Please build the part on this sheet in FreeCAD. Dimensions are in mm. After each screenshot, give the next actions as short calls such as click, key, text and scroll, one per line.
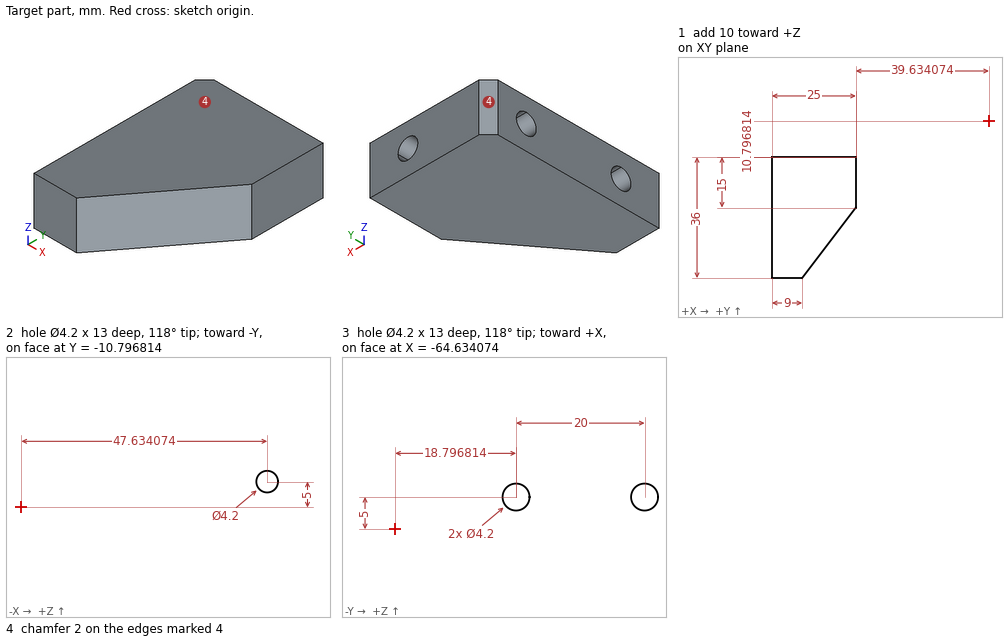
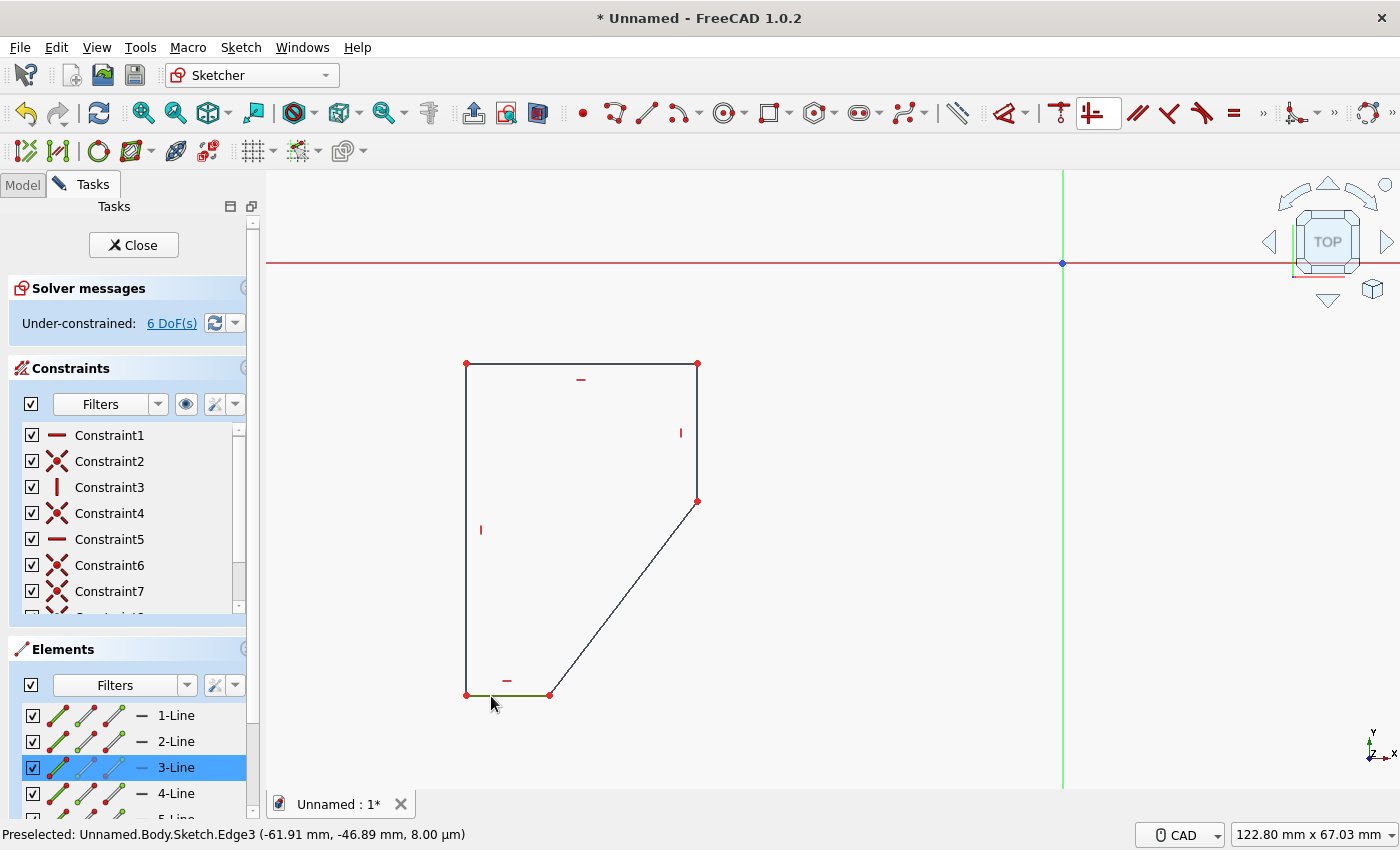
click(1028, 114)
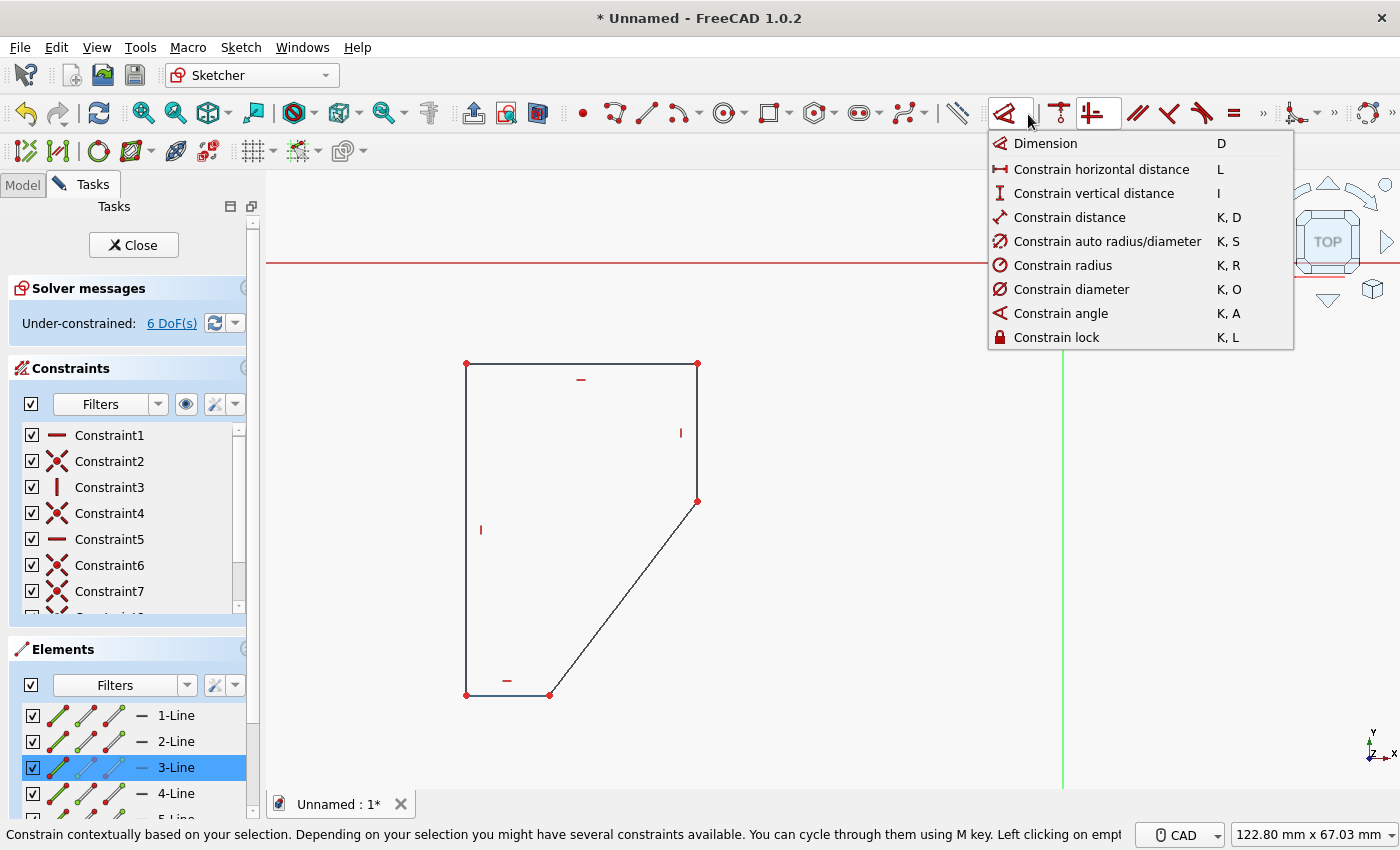
click(1141, 169)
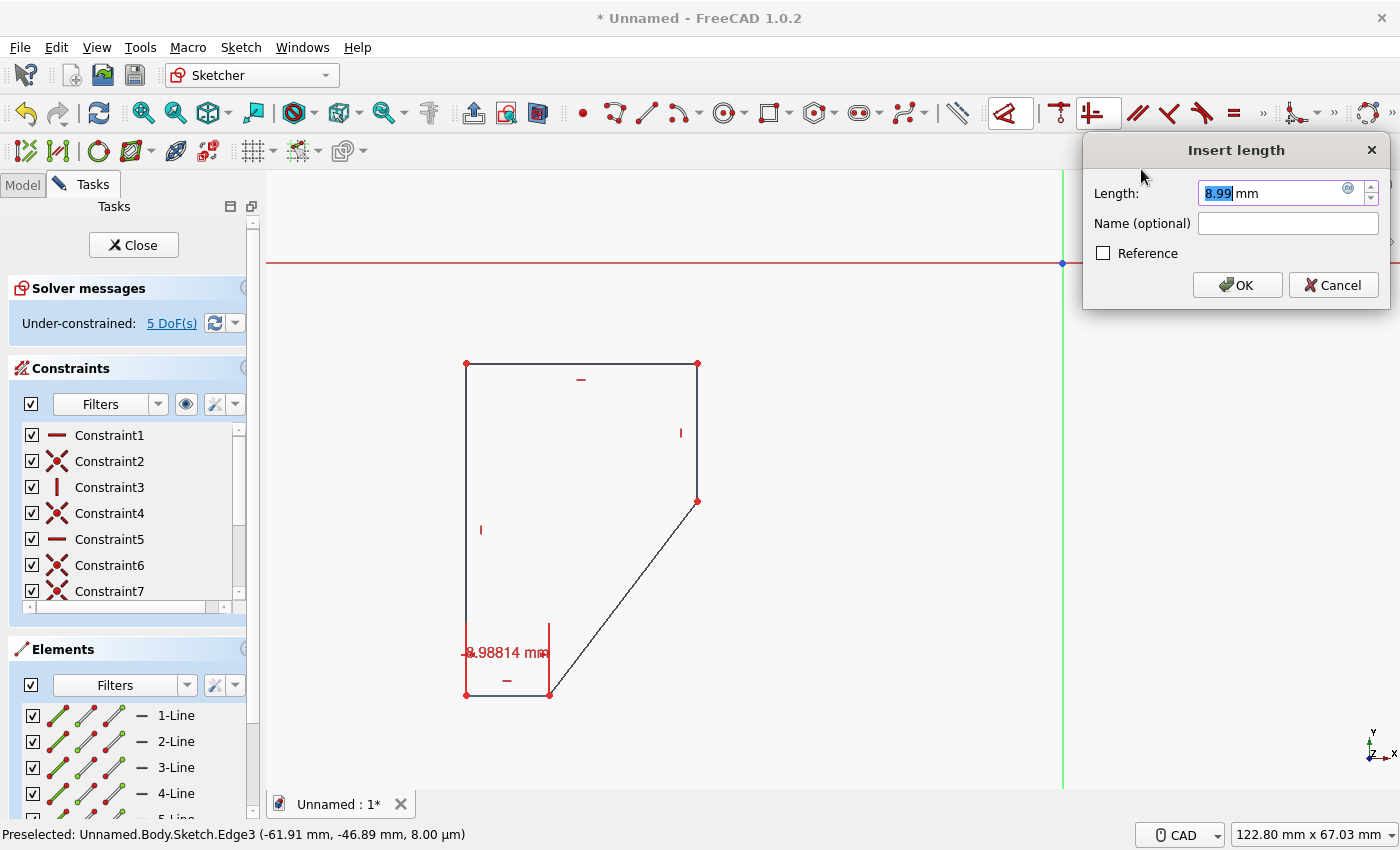
text(9)
key(Return)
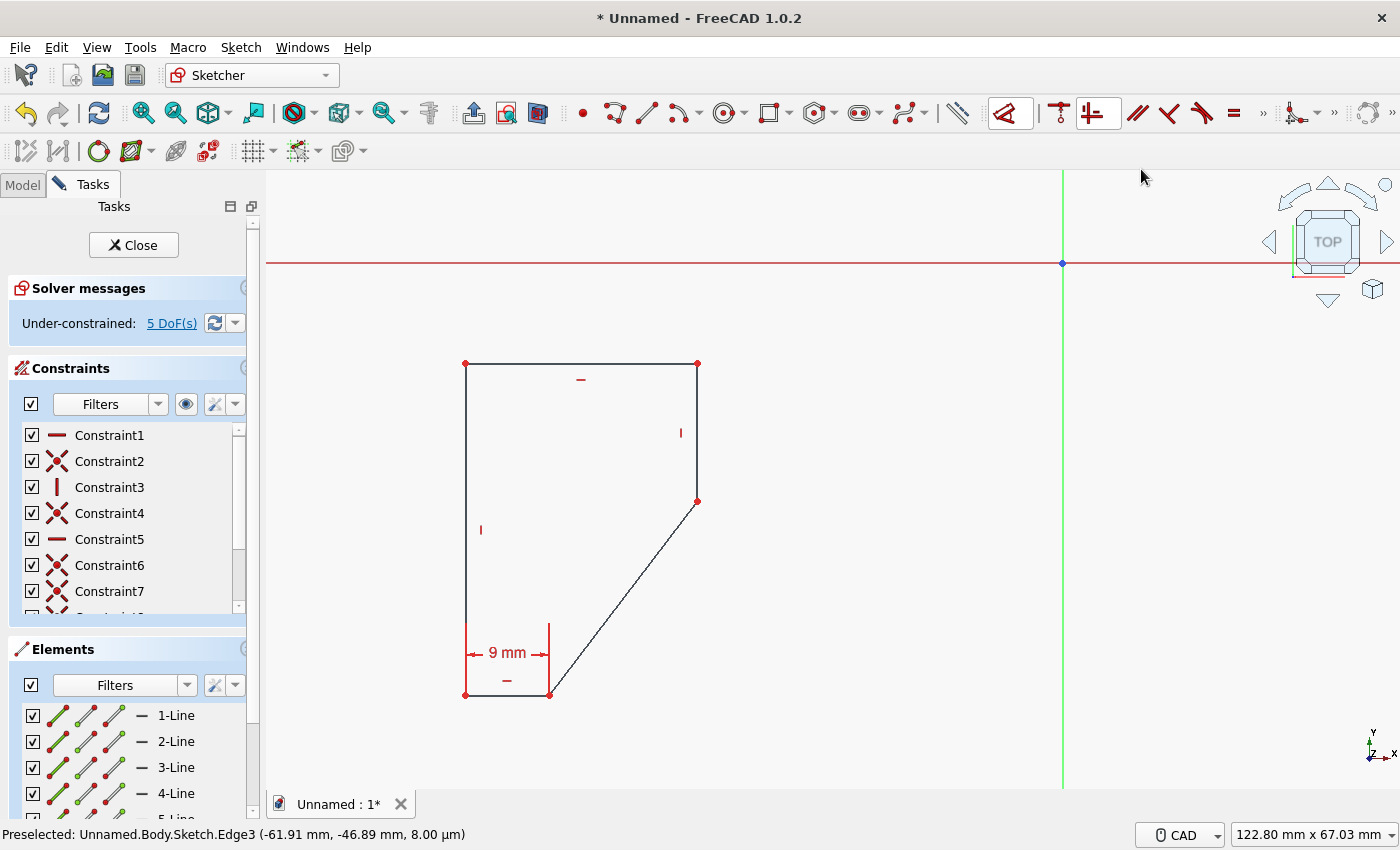
click(628, 364)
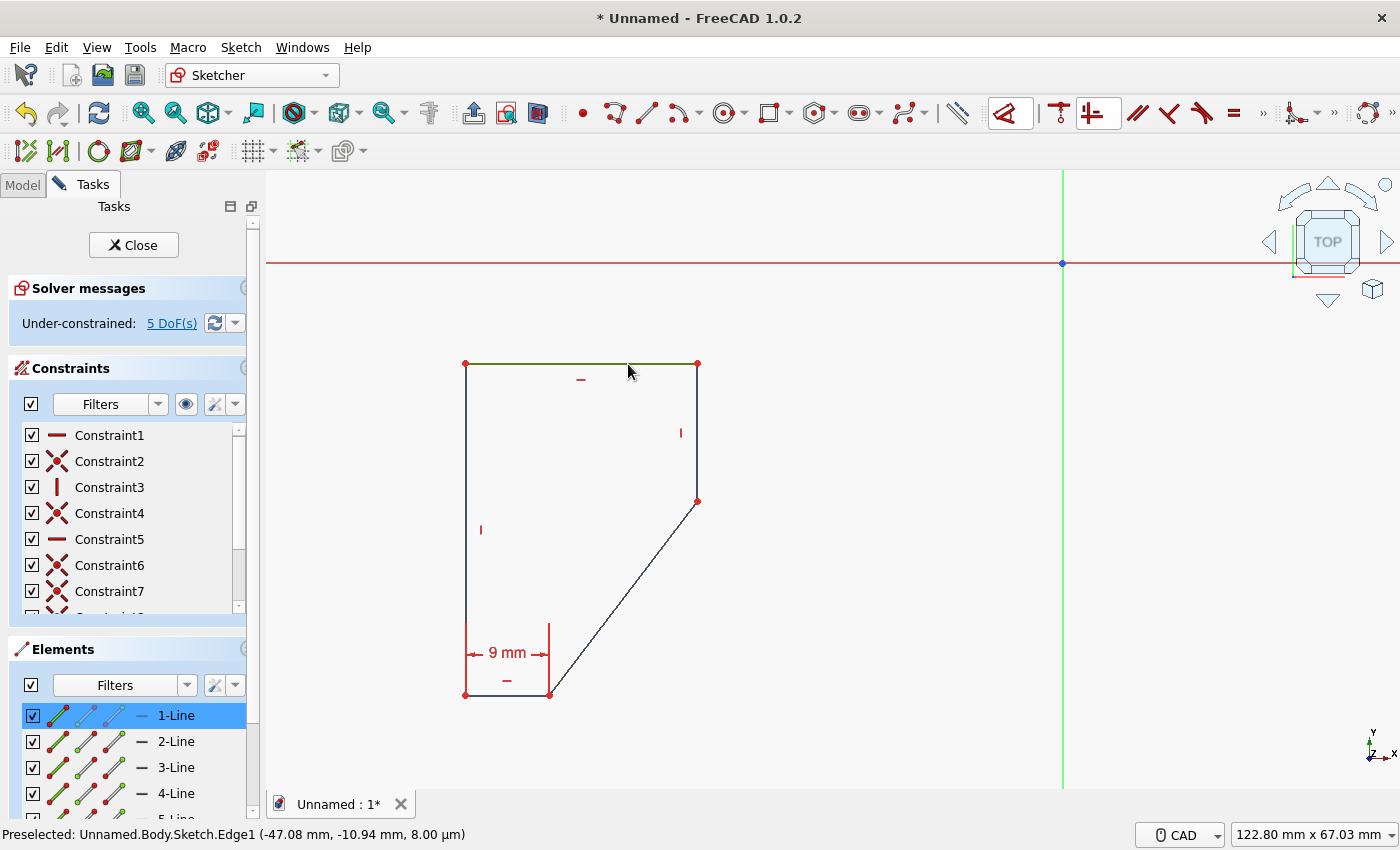
click(1028, 114)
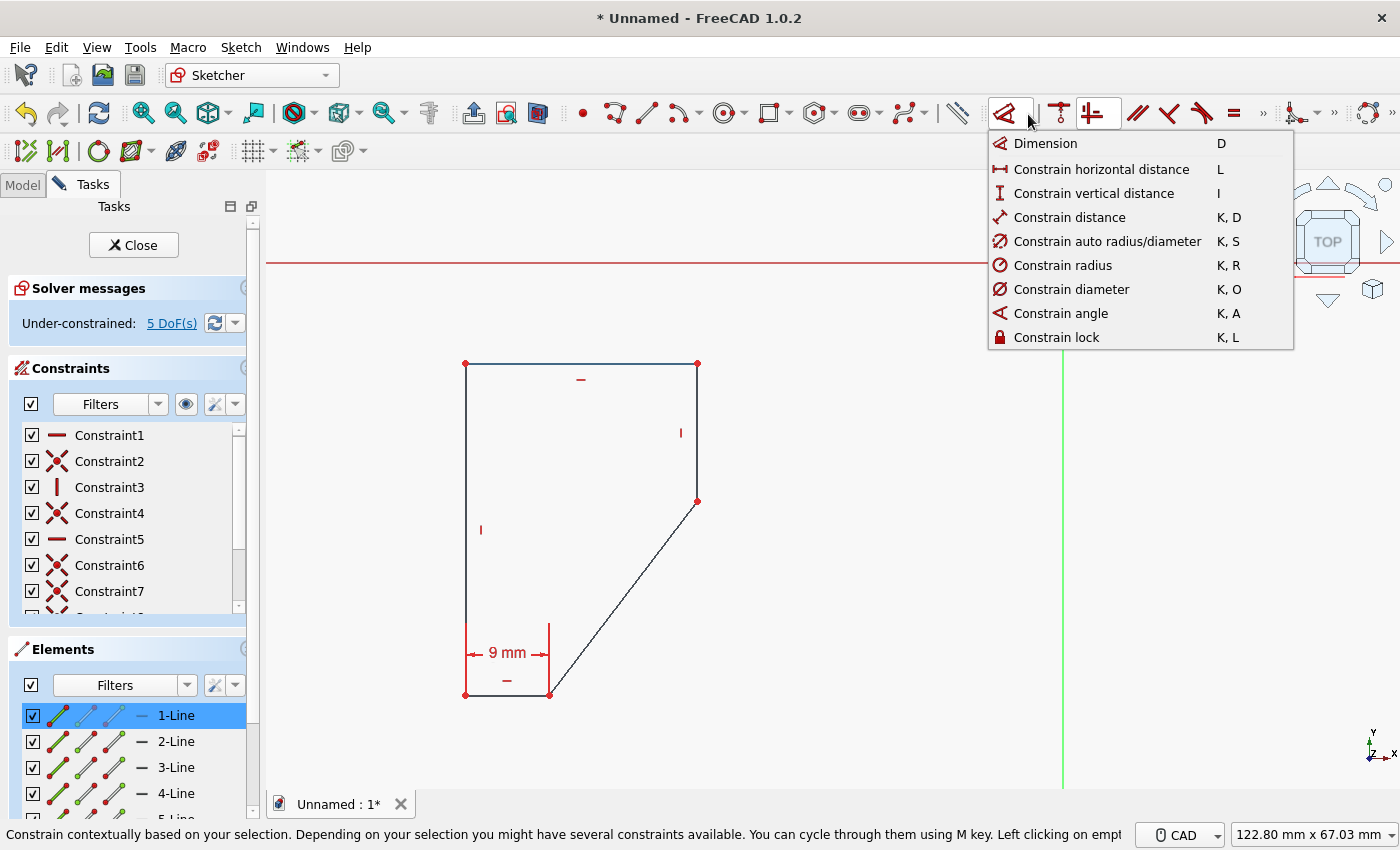
click(1141, 169)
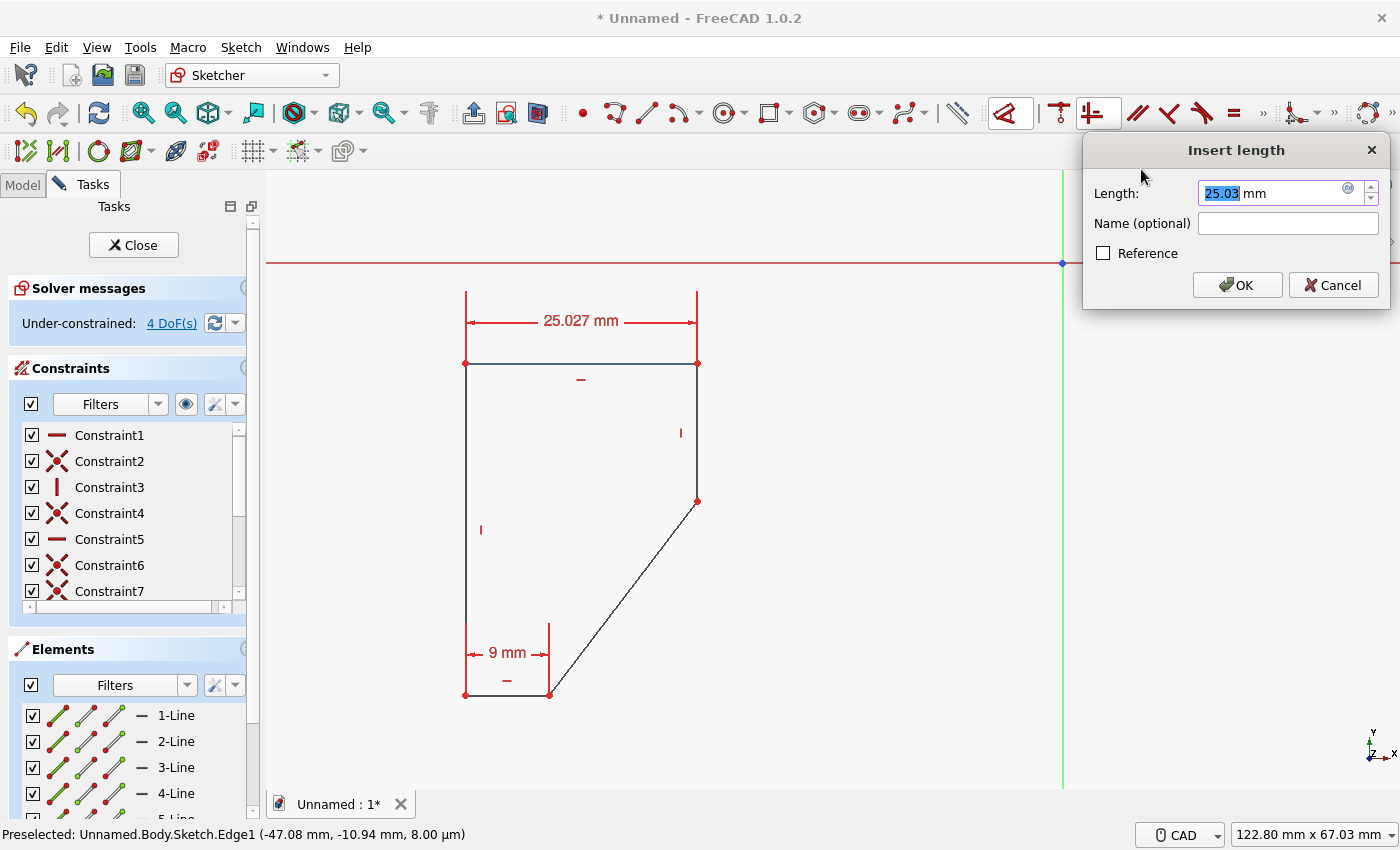
text(25)
key(Return)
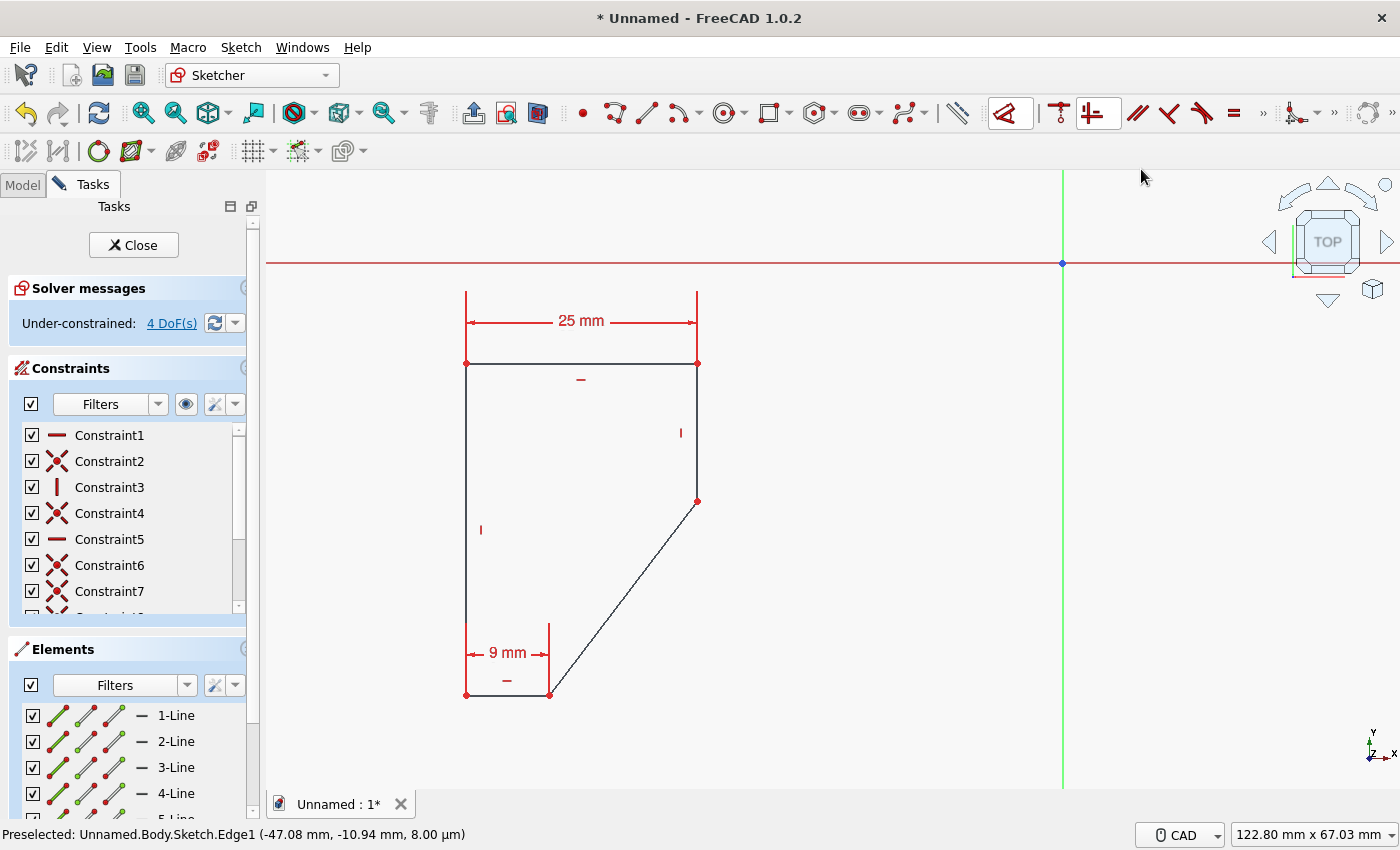
click(466, 464)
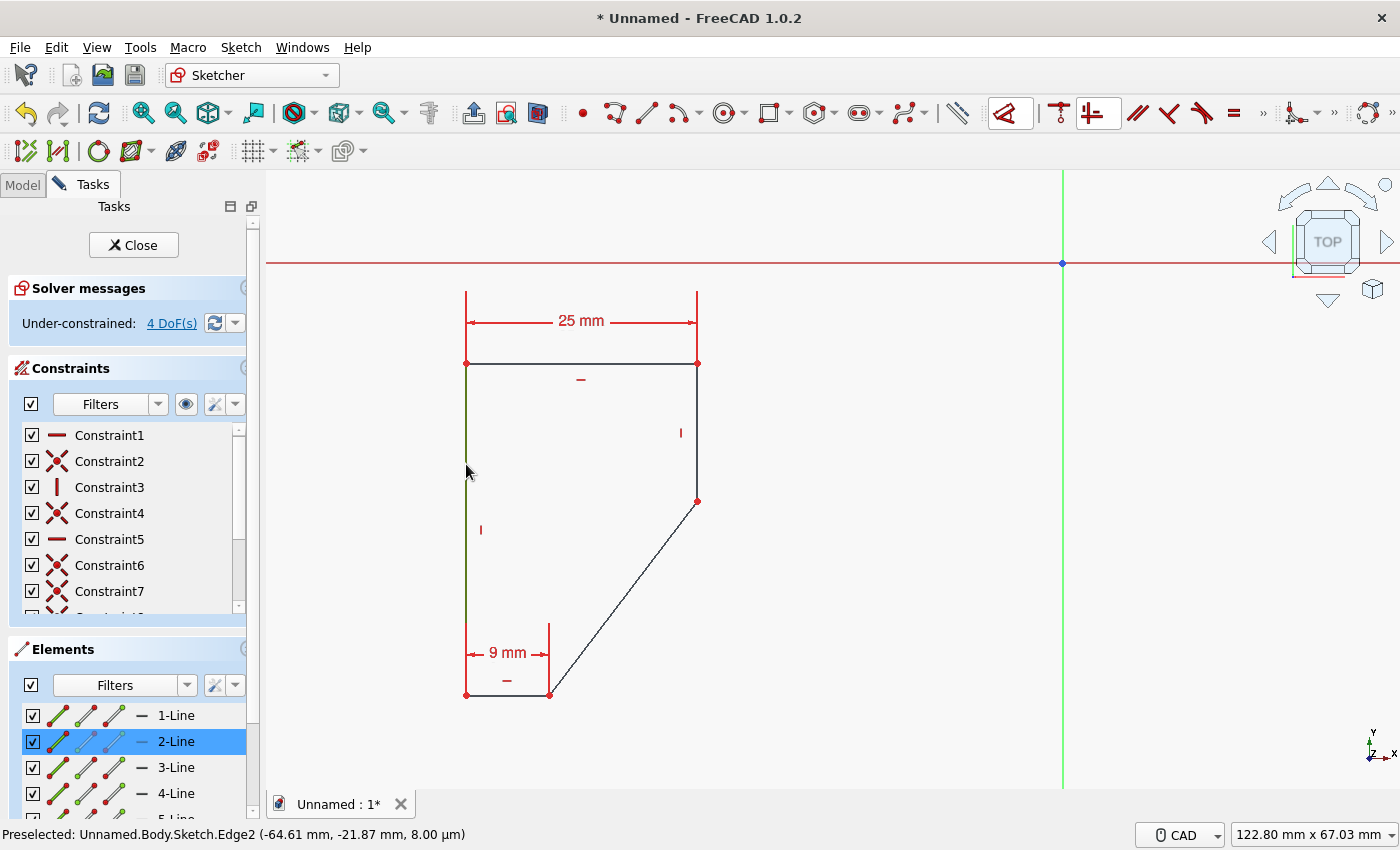
click(1028, 114)